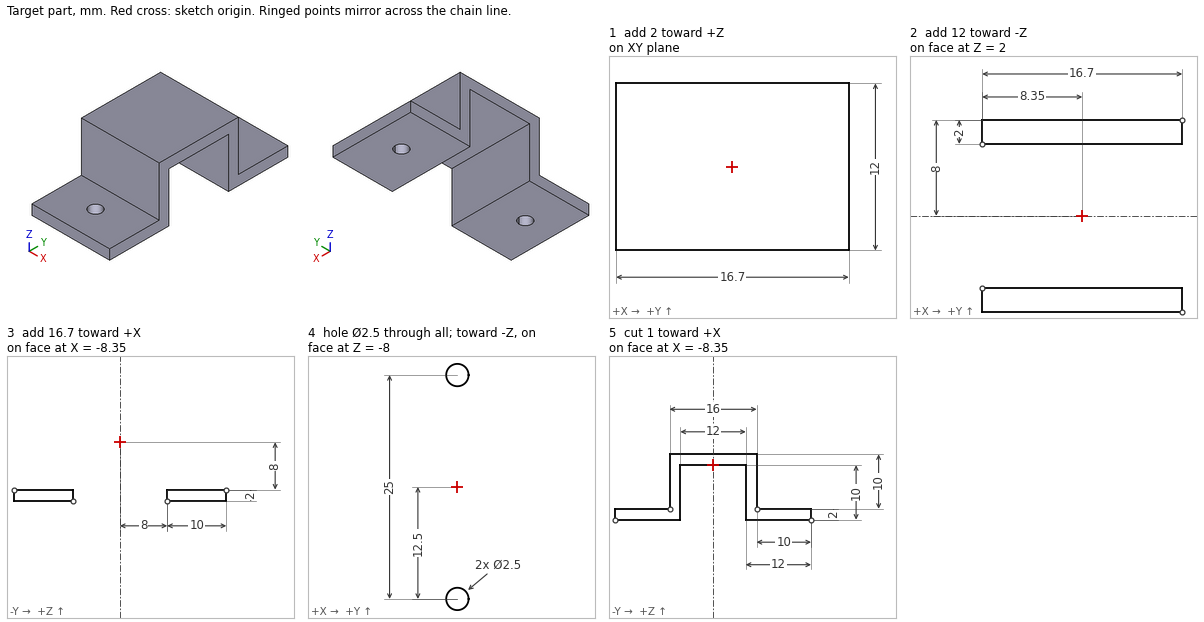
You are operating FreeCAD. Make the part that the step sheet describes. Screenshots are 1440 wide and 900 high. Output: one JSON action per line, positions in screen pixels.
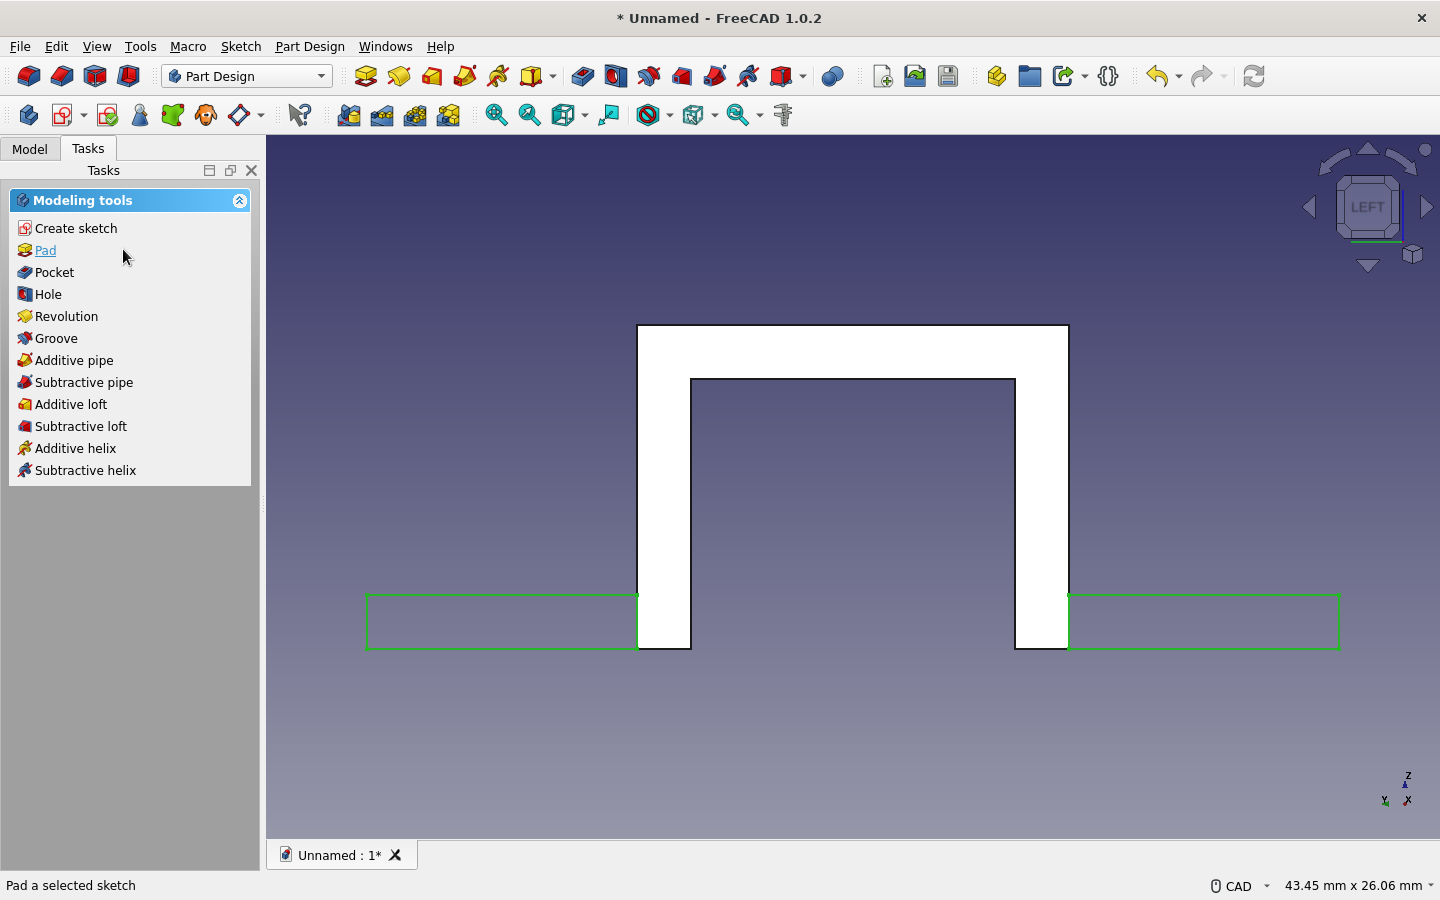
{"action": "left_click", "coordinate": [366, 76]}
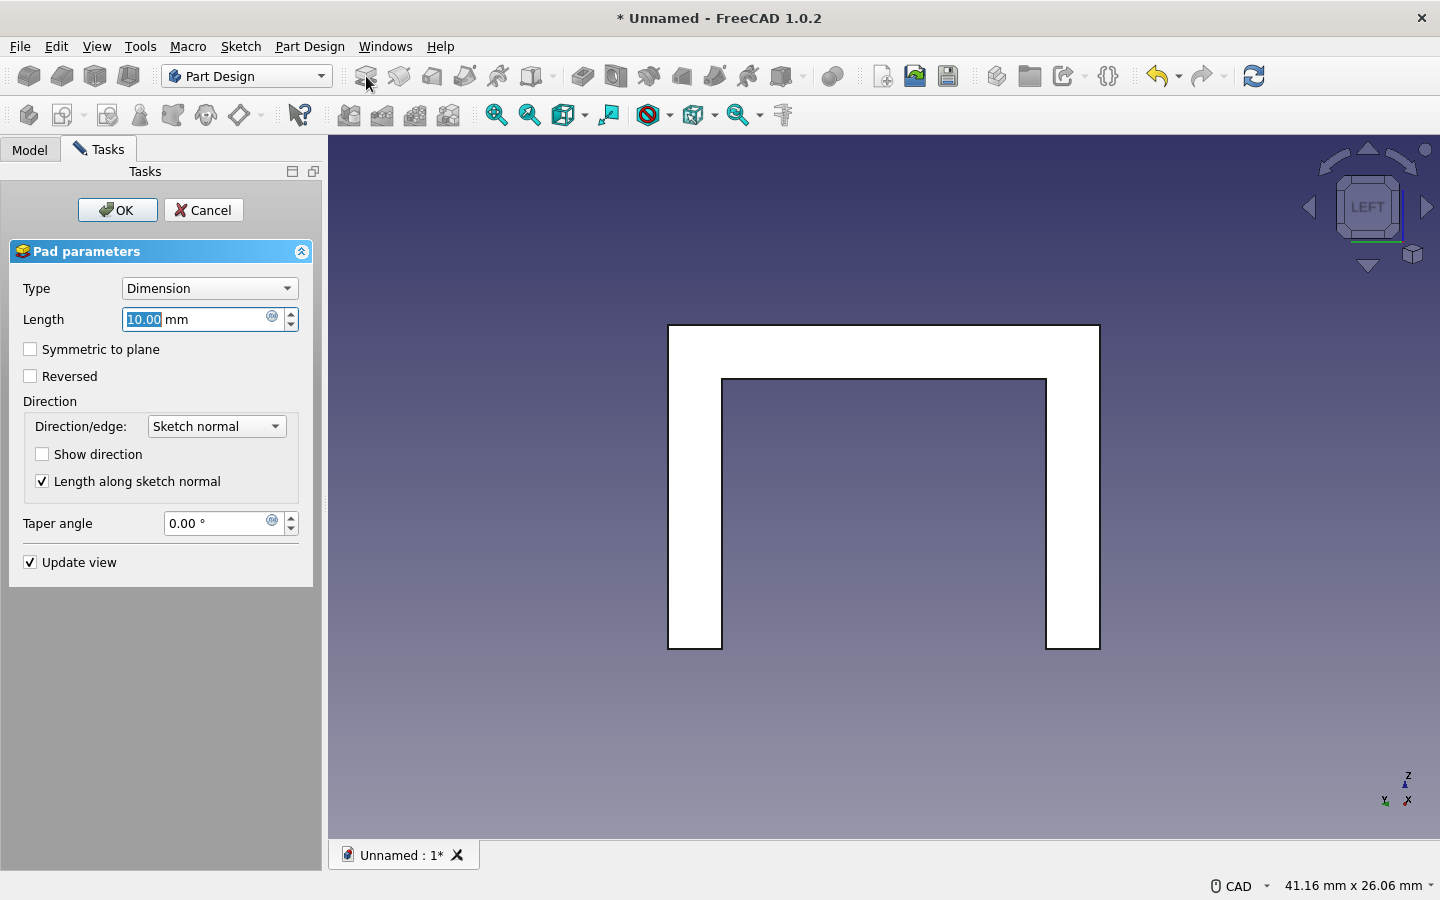
{"action": "type", "text": "16.7"}
{"action": "key", "text": "Tab"}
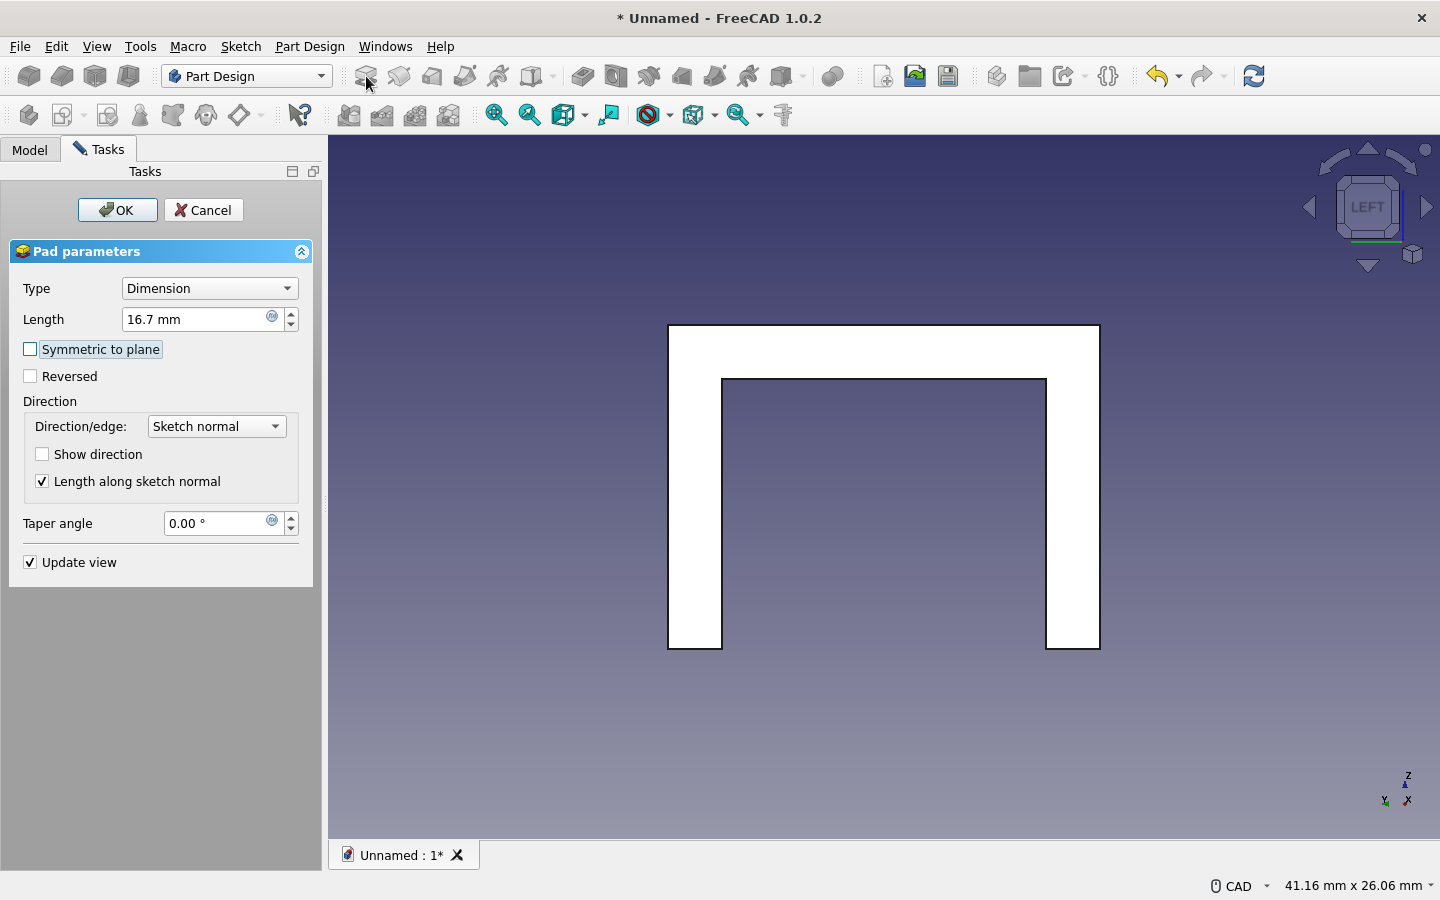
{"action": "left_click", "coordinate": [31, 376]}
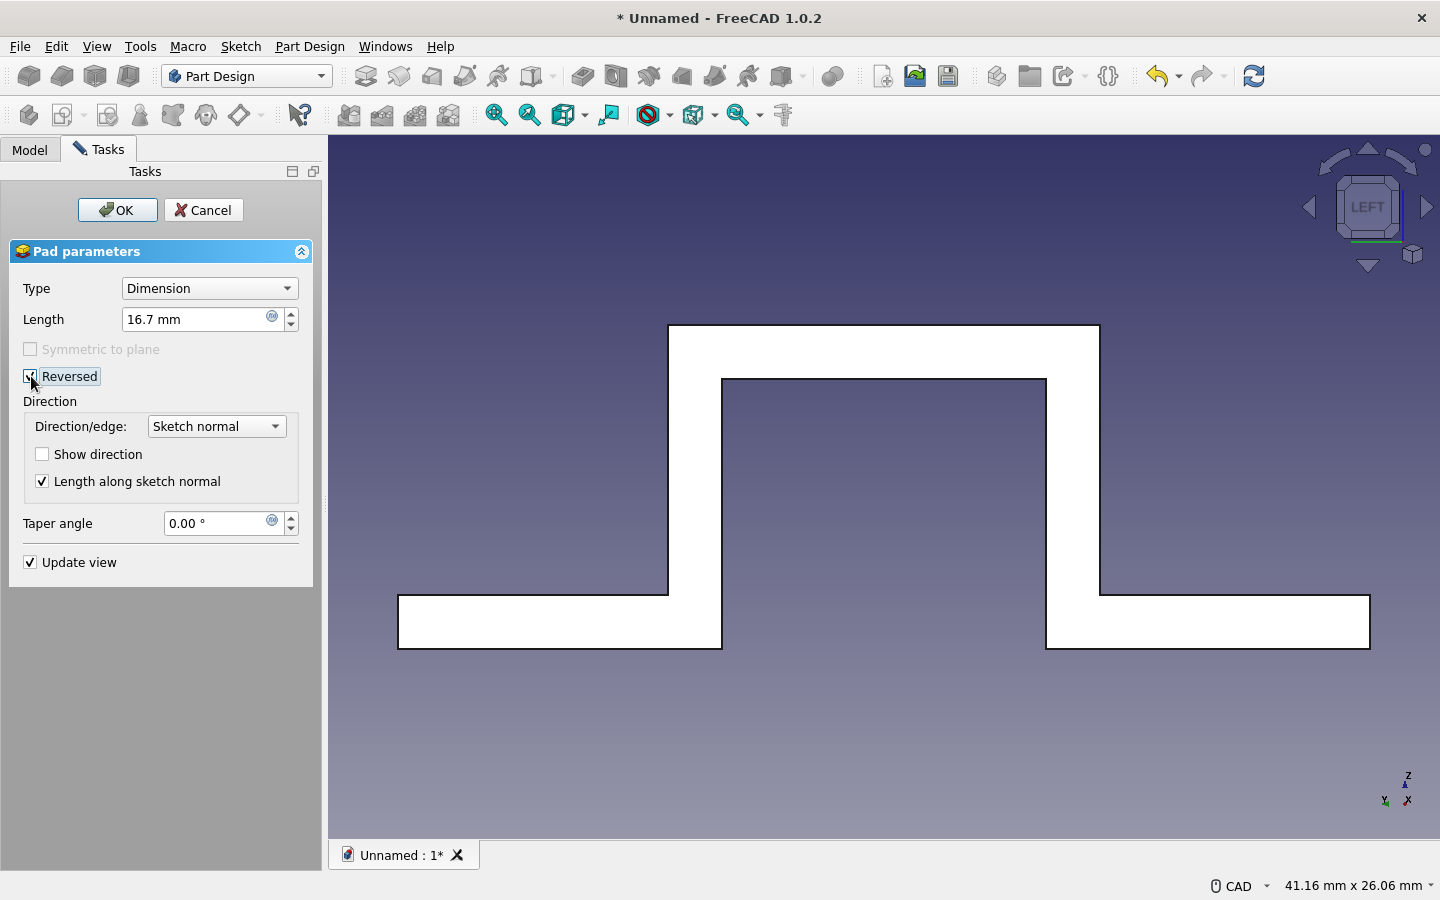
{"action": "left_click", "coordinate": [118, 210]}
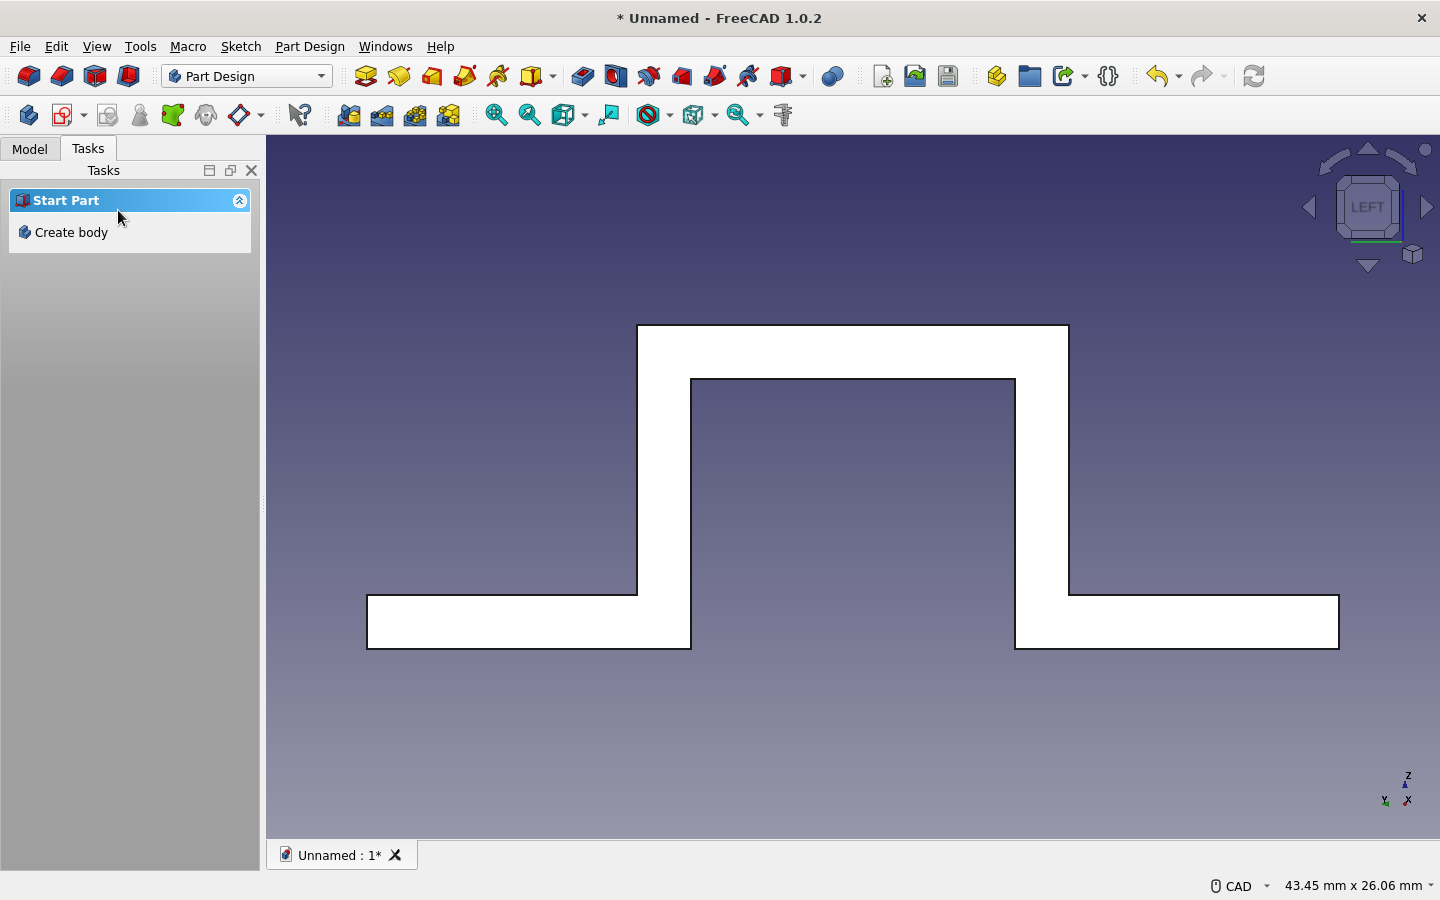
{"action": "key", "text": "0"}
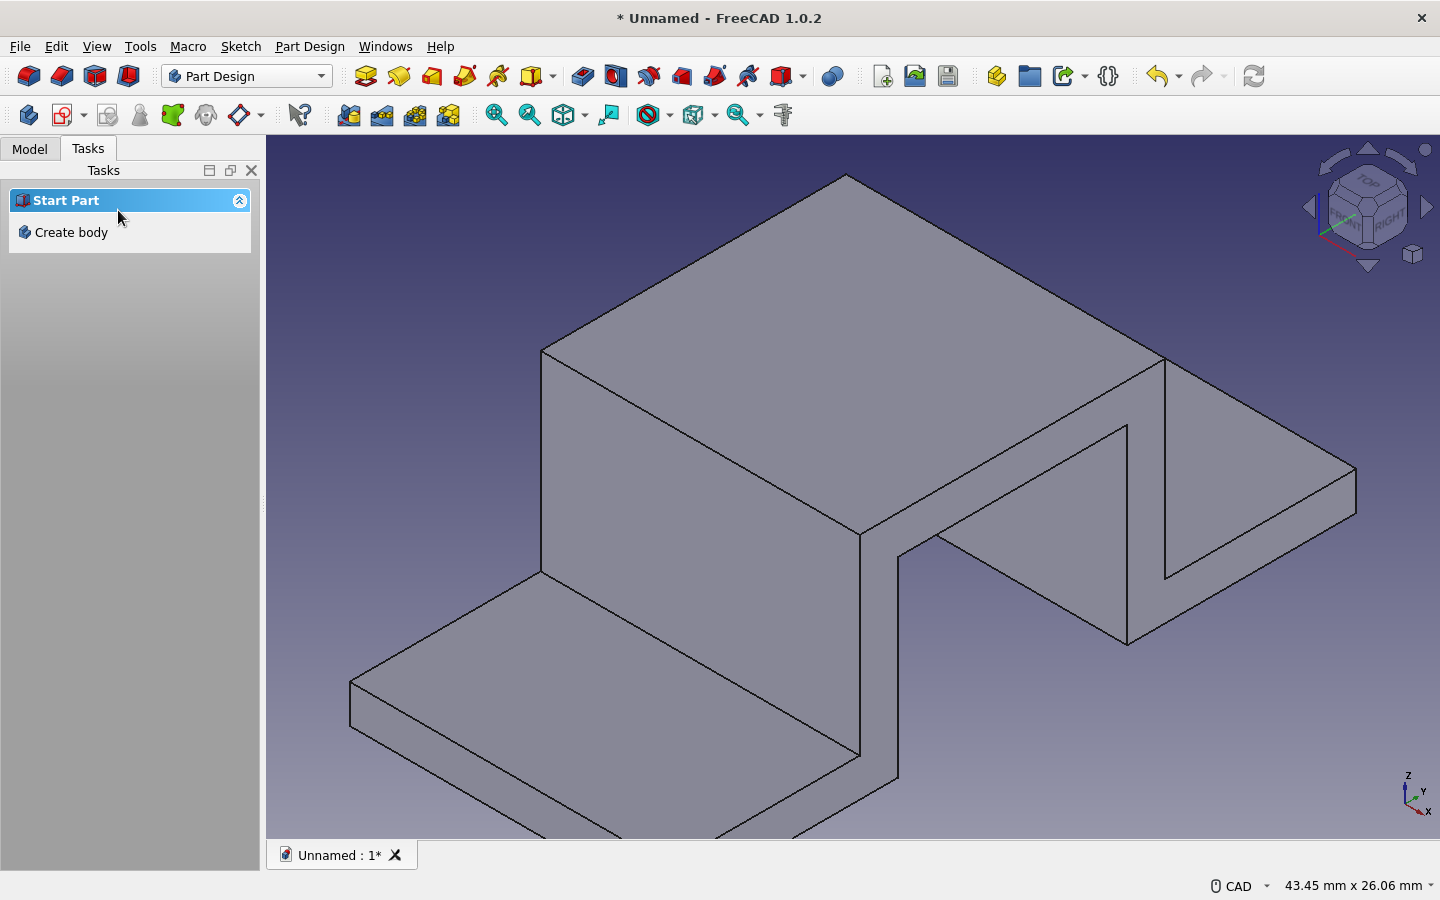
{"action": "key", "text": "v f"}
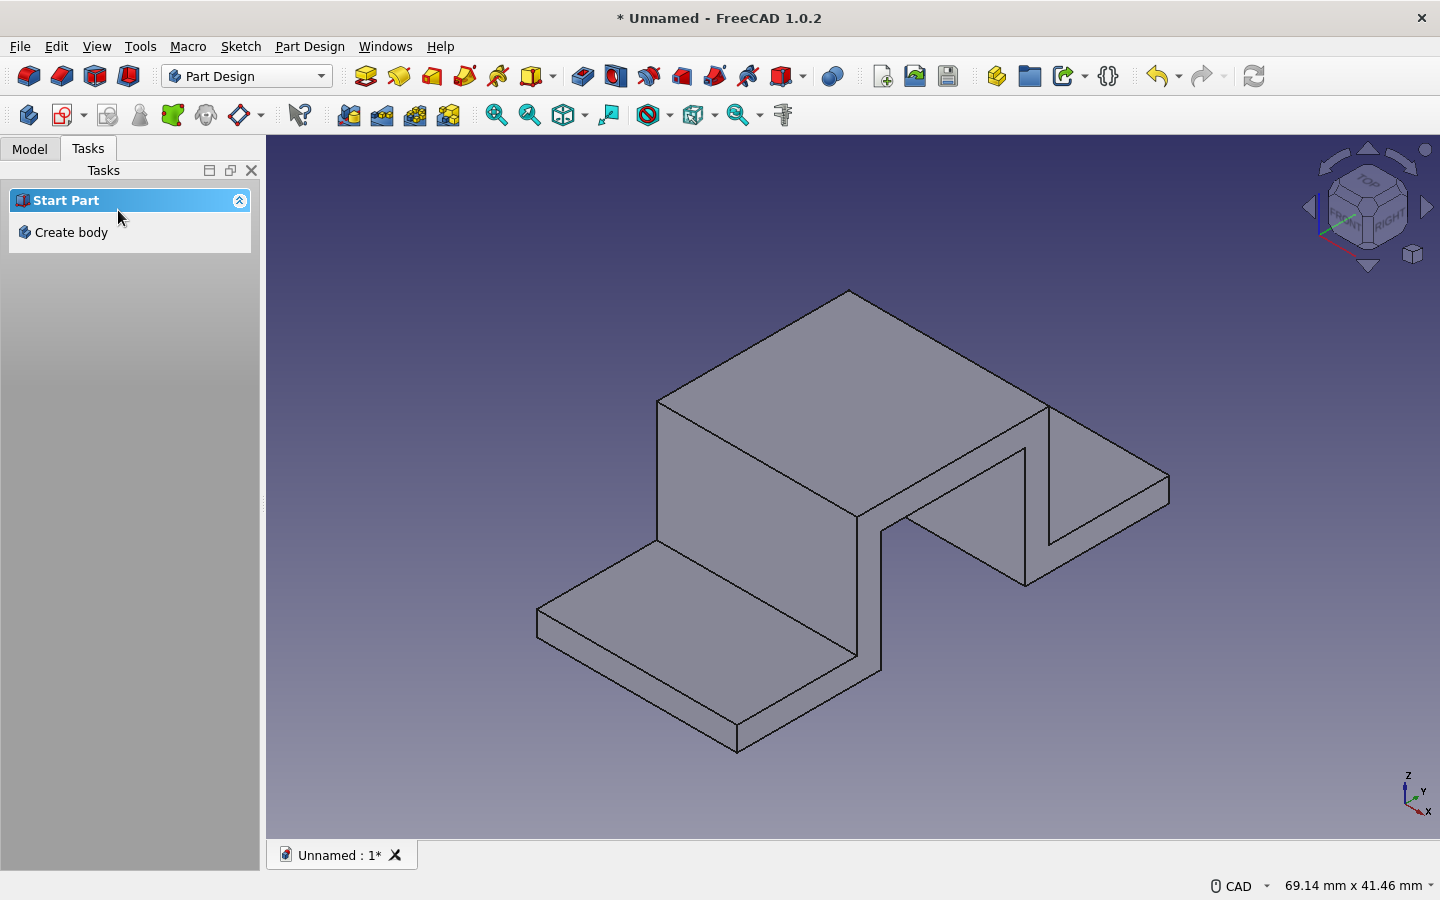
{"action": "left_click", "coordinate": [726, 648]}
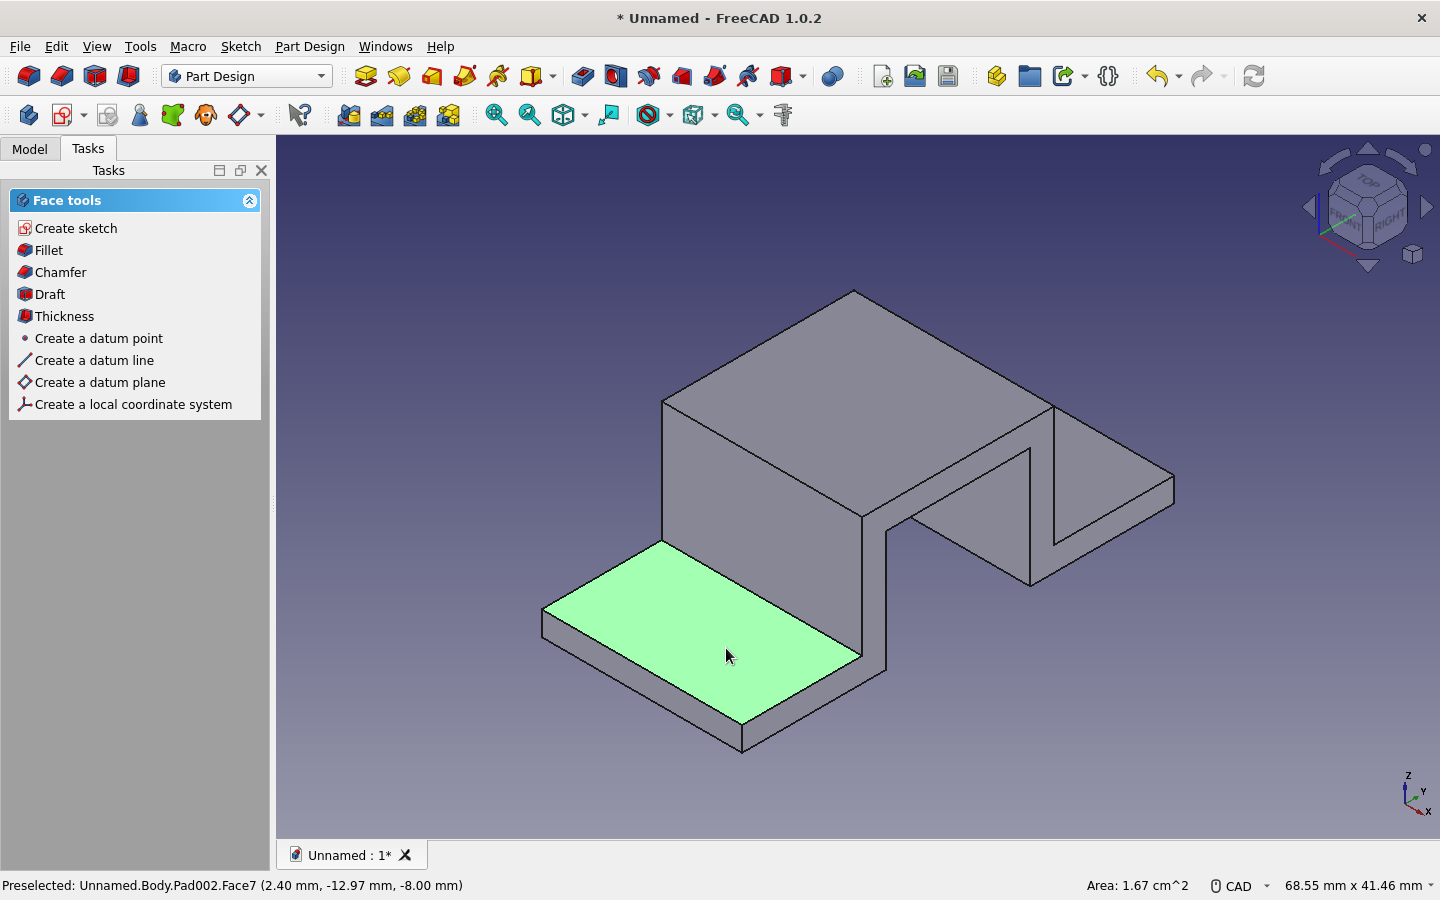
{"action": "left_click", "coordinate": [62, 116]}